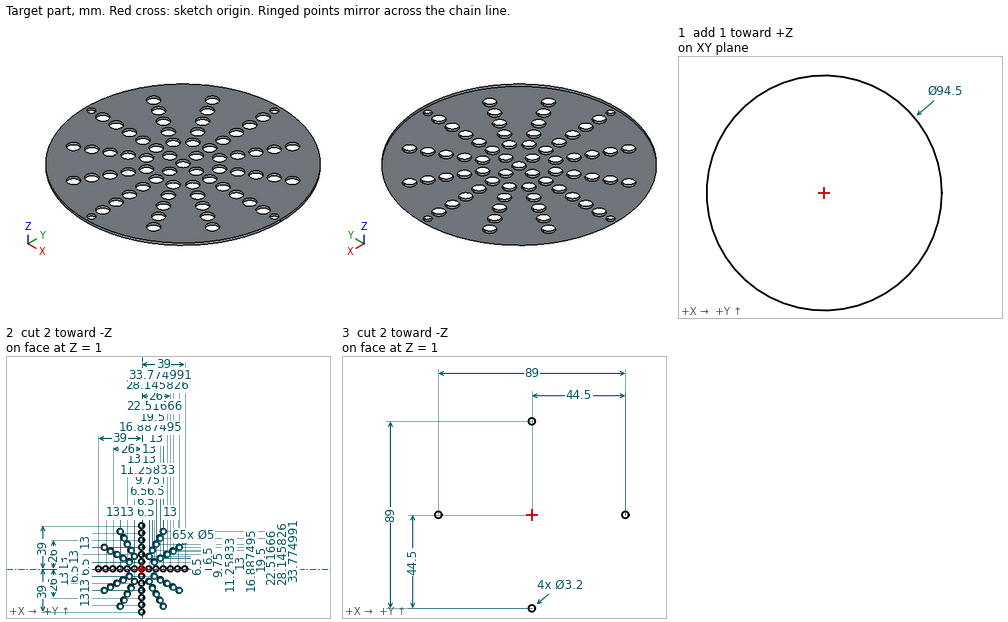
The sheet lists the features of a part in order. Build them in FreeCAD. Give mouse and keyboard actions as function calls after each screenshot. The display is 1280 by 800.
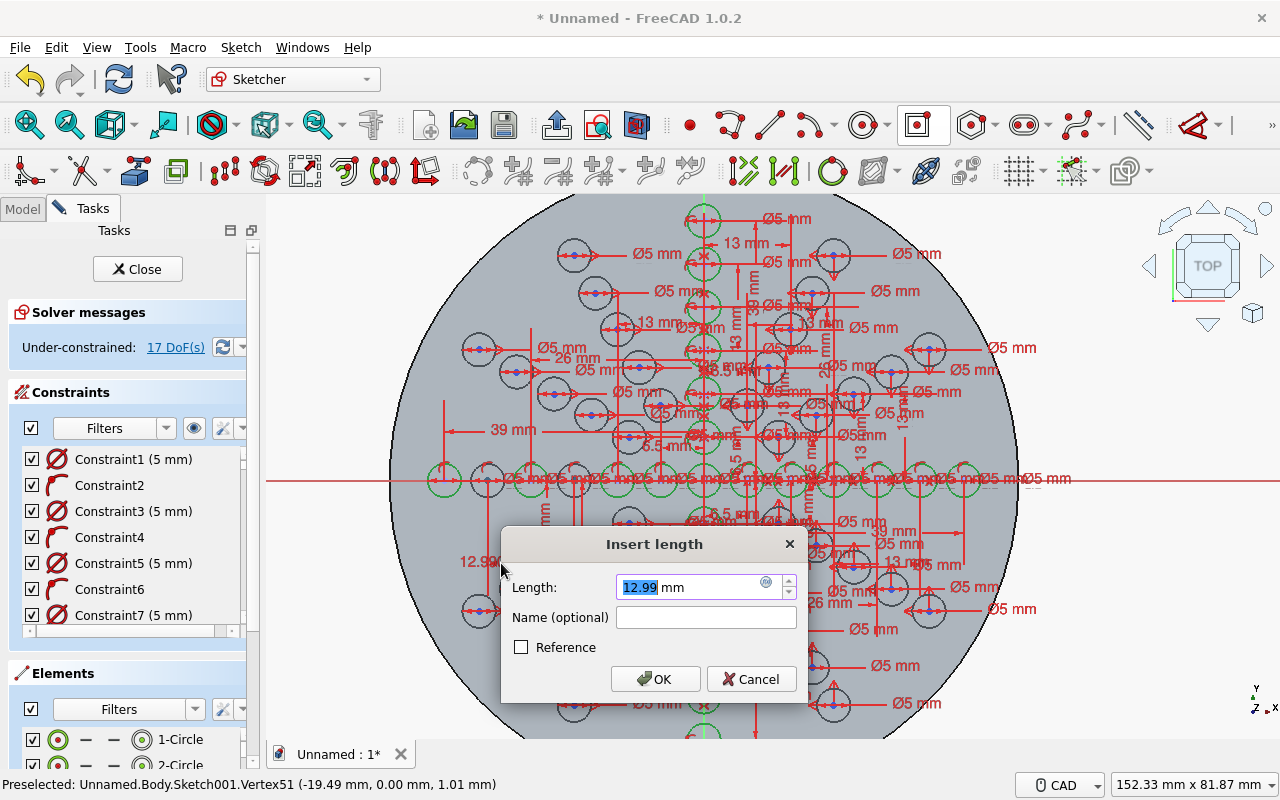
text(13)
key(Return)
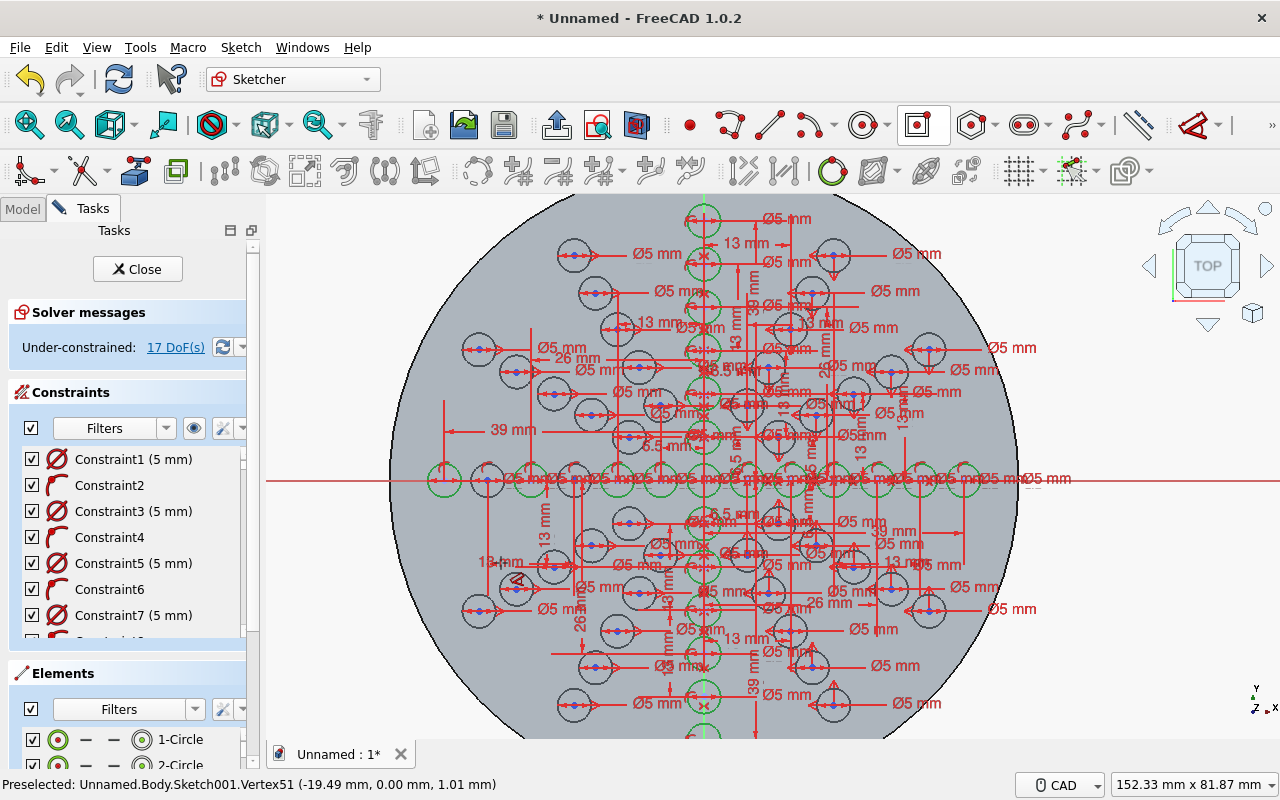
click(661, 555)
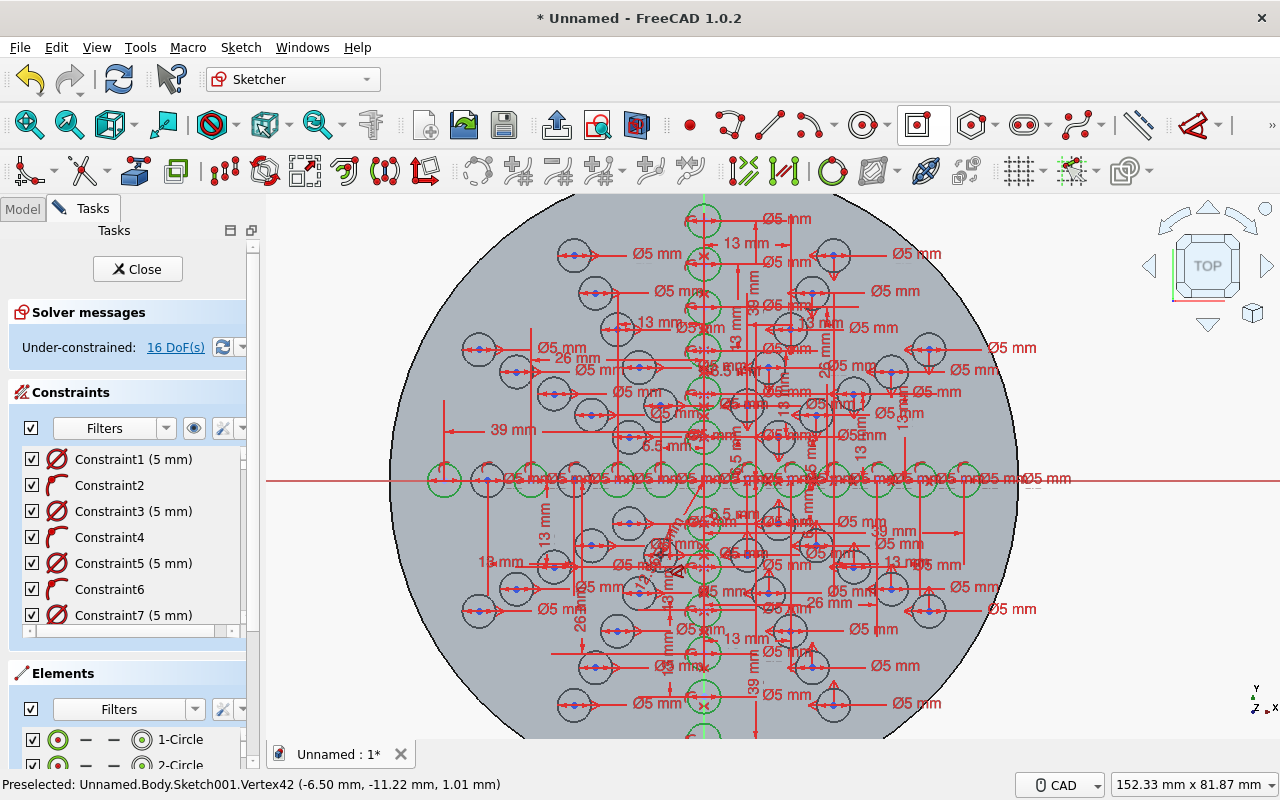
click(574, 481)
click(587, 447)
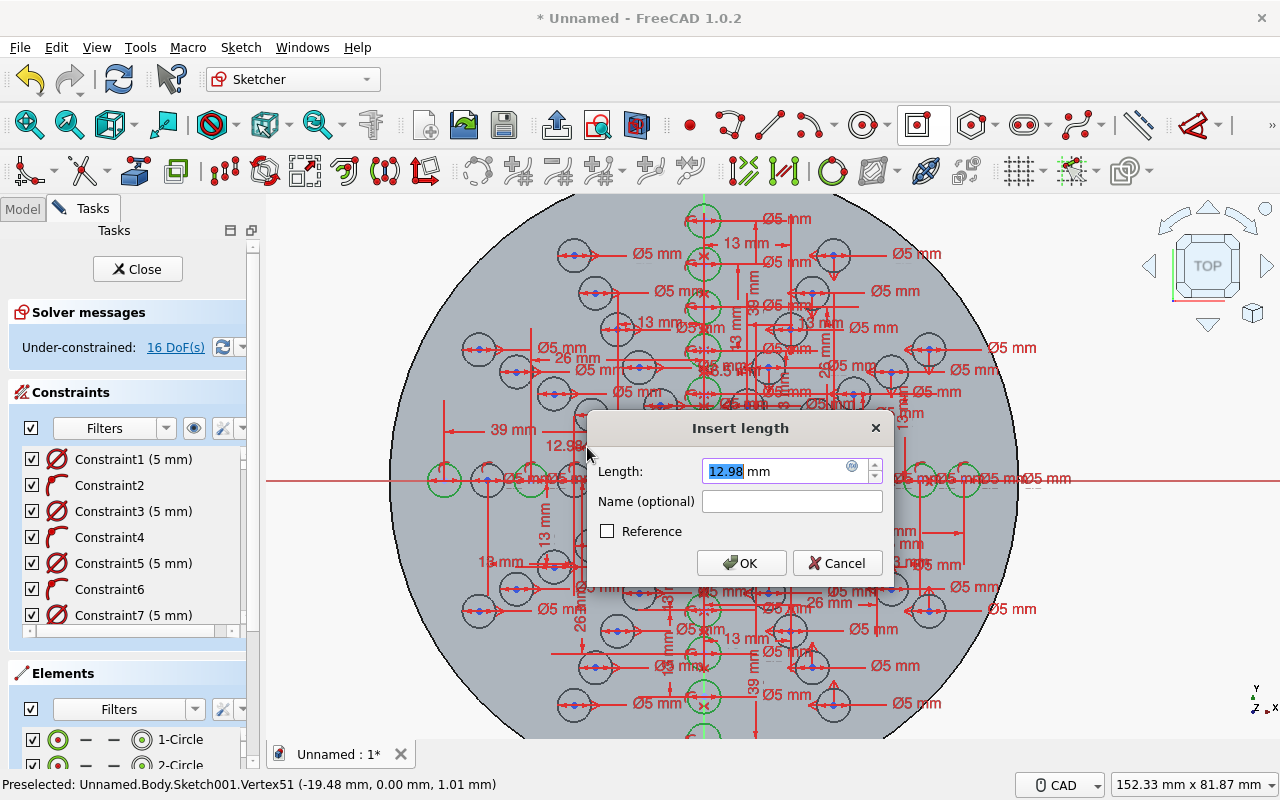
text(13)
key(Return)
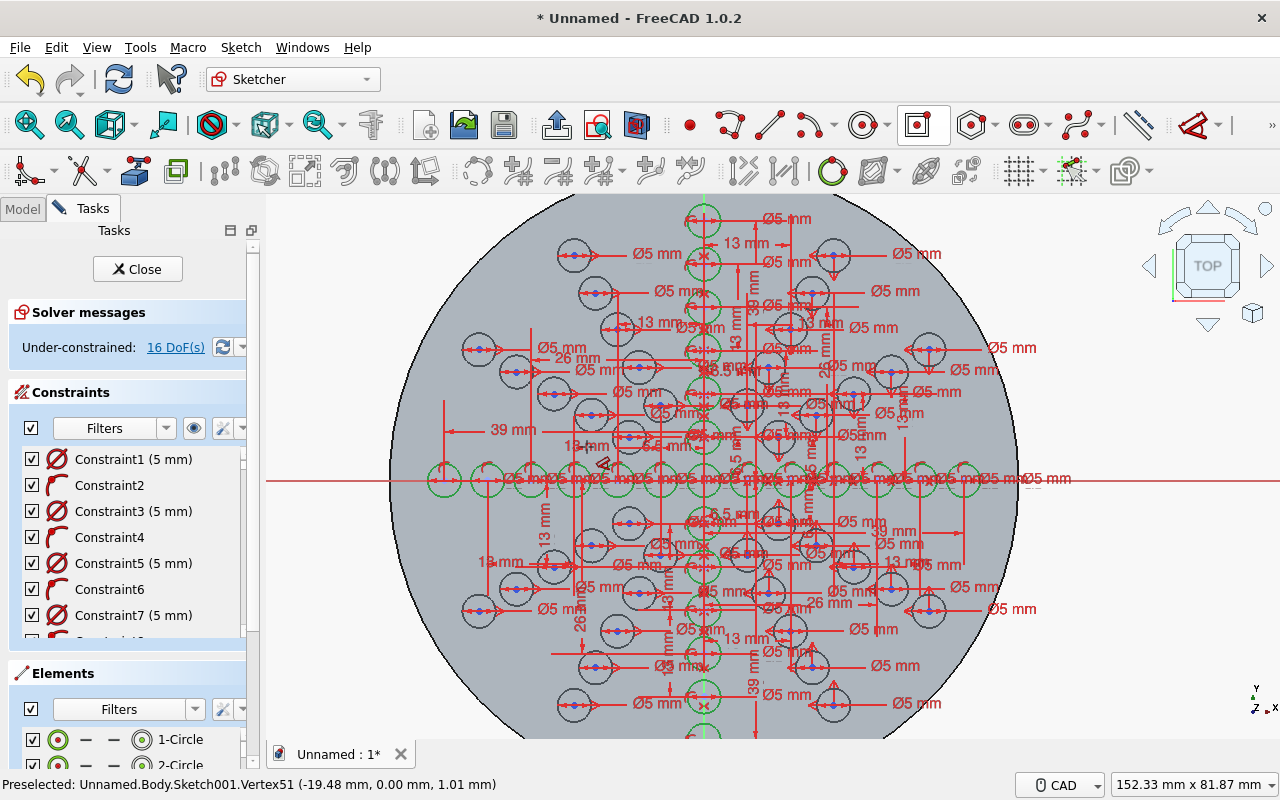
click(834, 256)
click(739, 611)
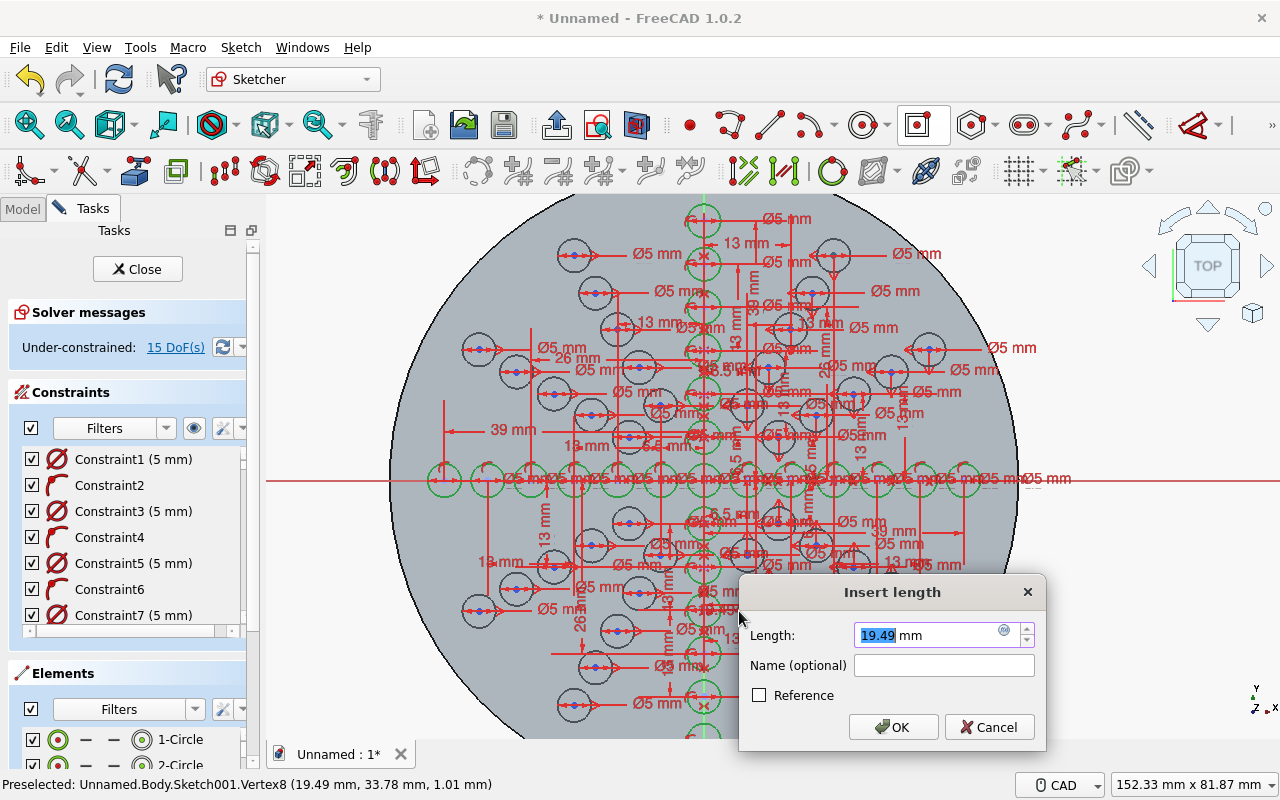
text(19.5)
key(Return)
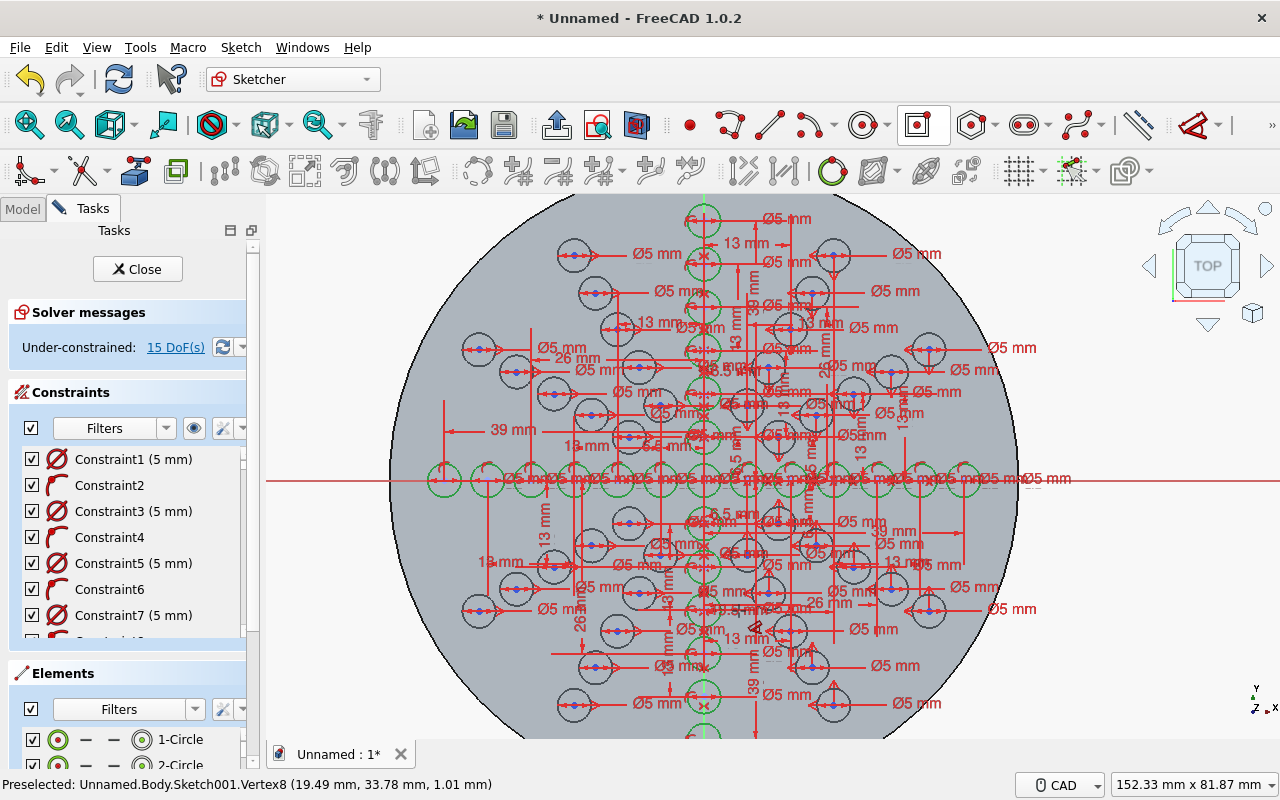
click(769, 368)
click(736, 310)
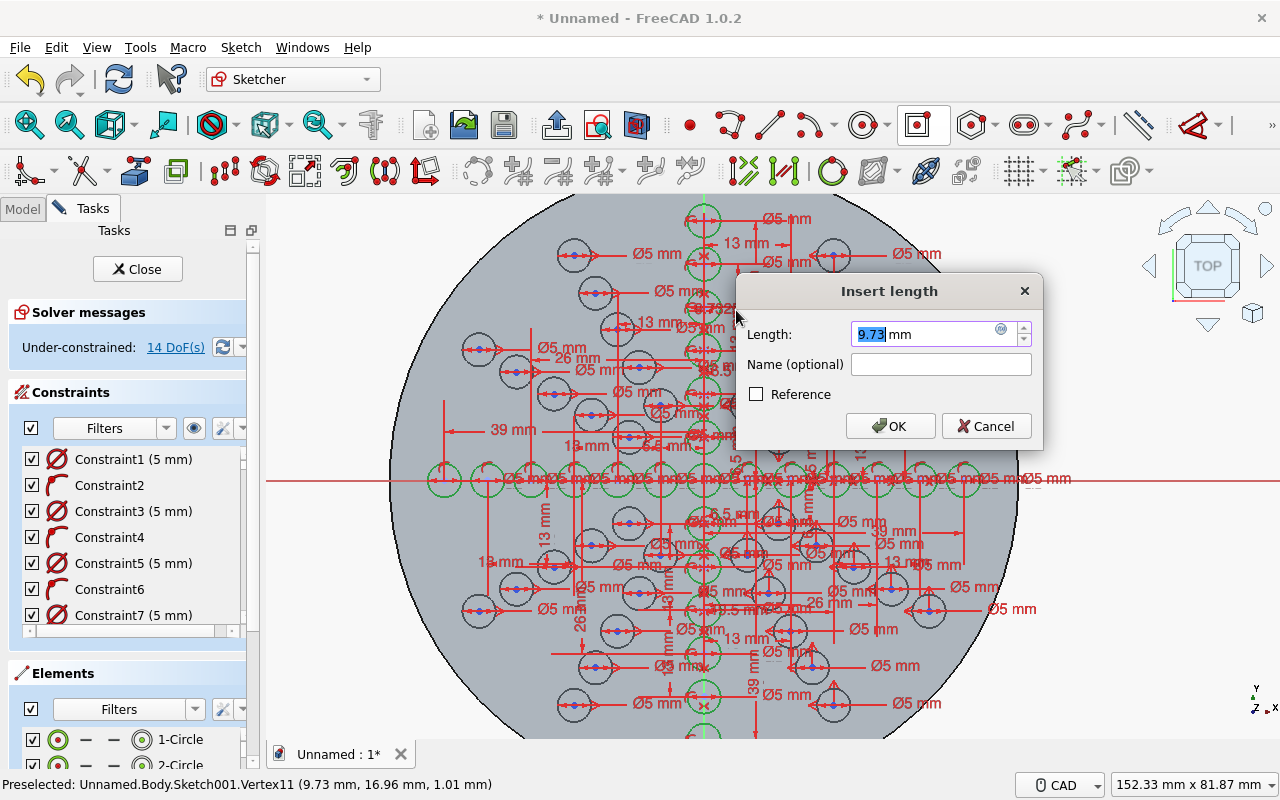
text(9.75)
key(Return)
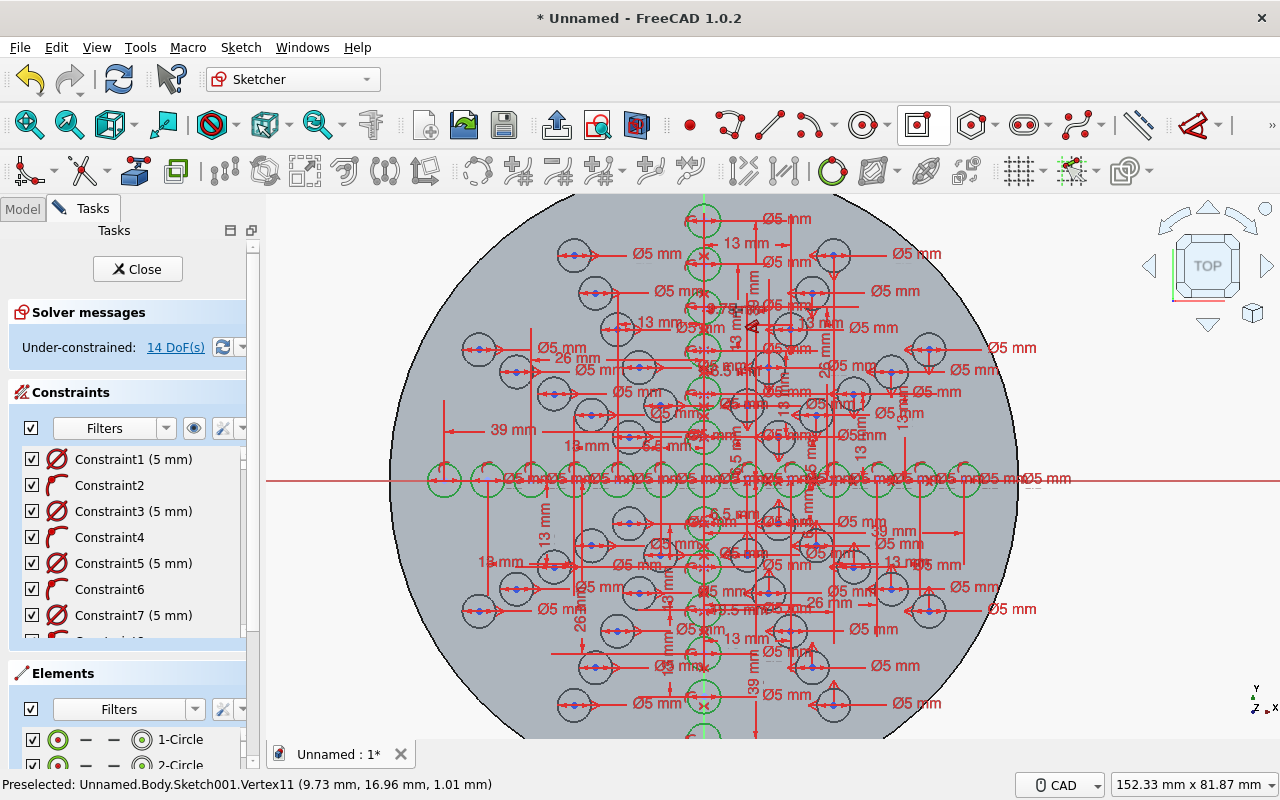
click(929, 350)
click(963, 385)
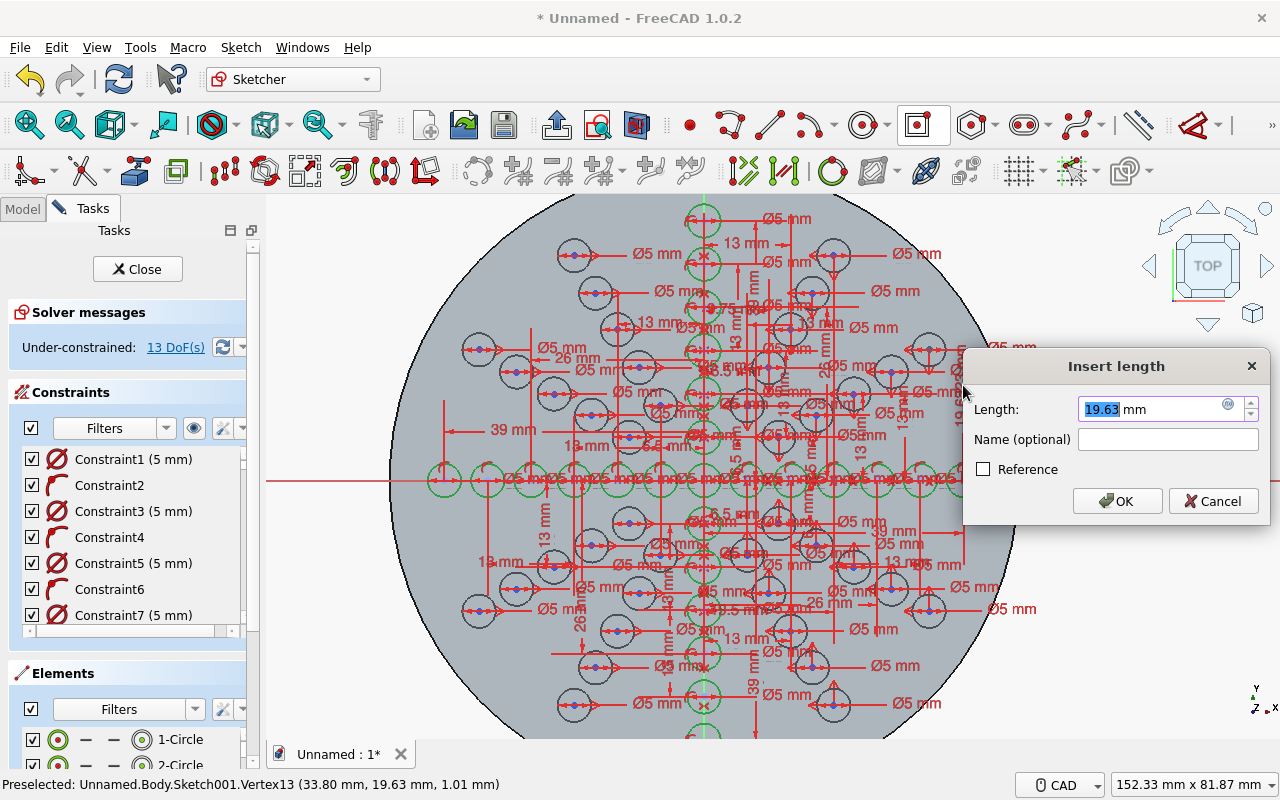
text(19.5)
key(Return)